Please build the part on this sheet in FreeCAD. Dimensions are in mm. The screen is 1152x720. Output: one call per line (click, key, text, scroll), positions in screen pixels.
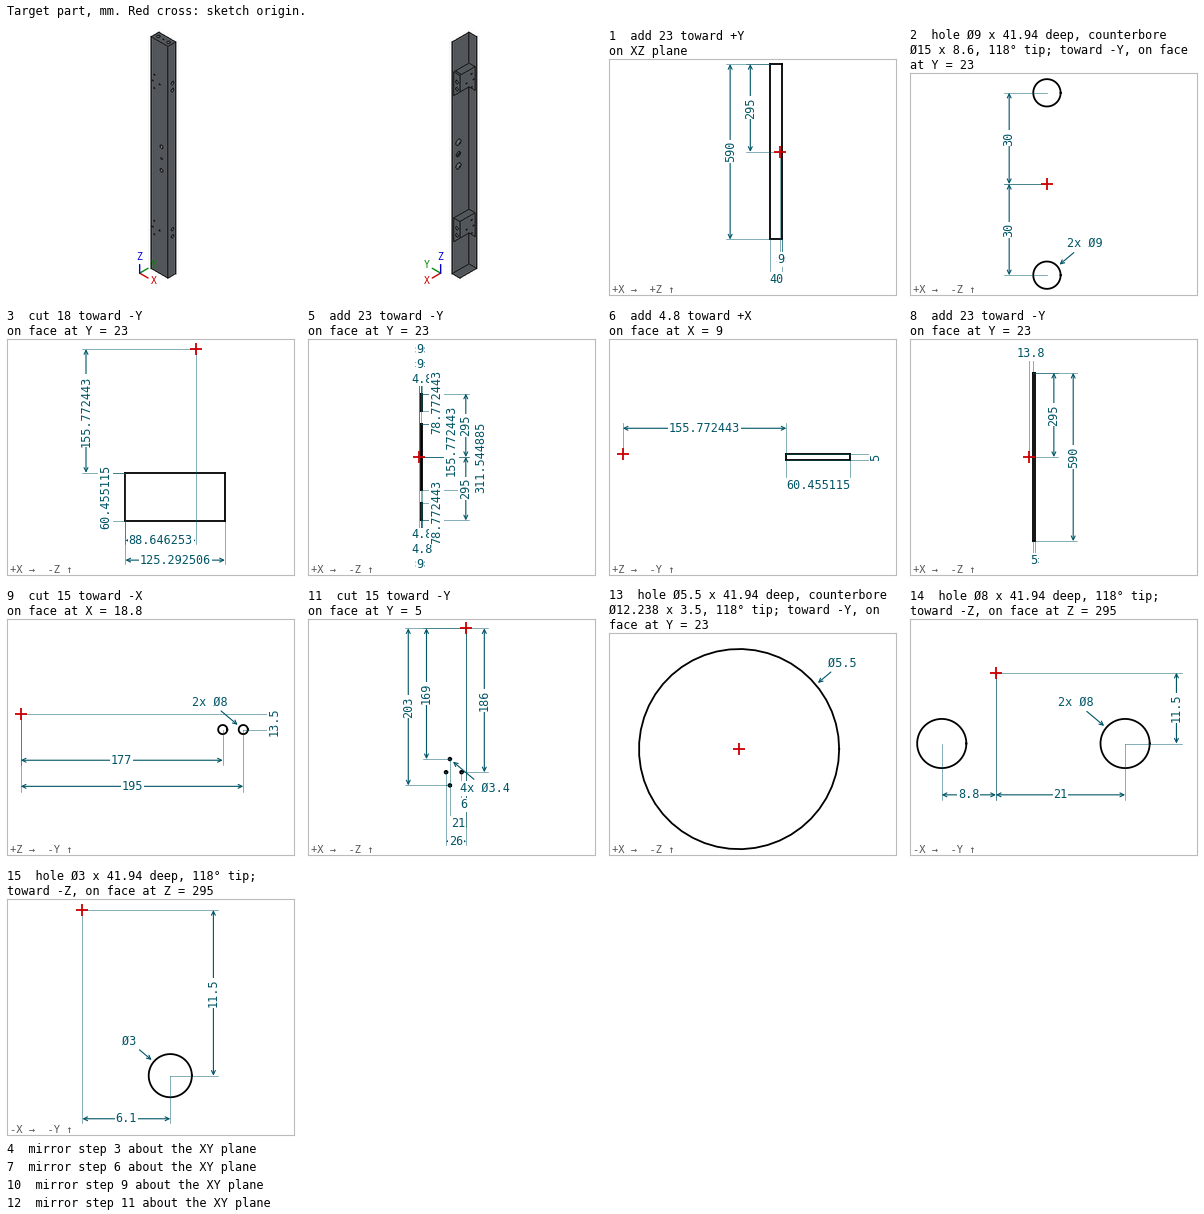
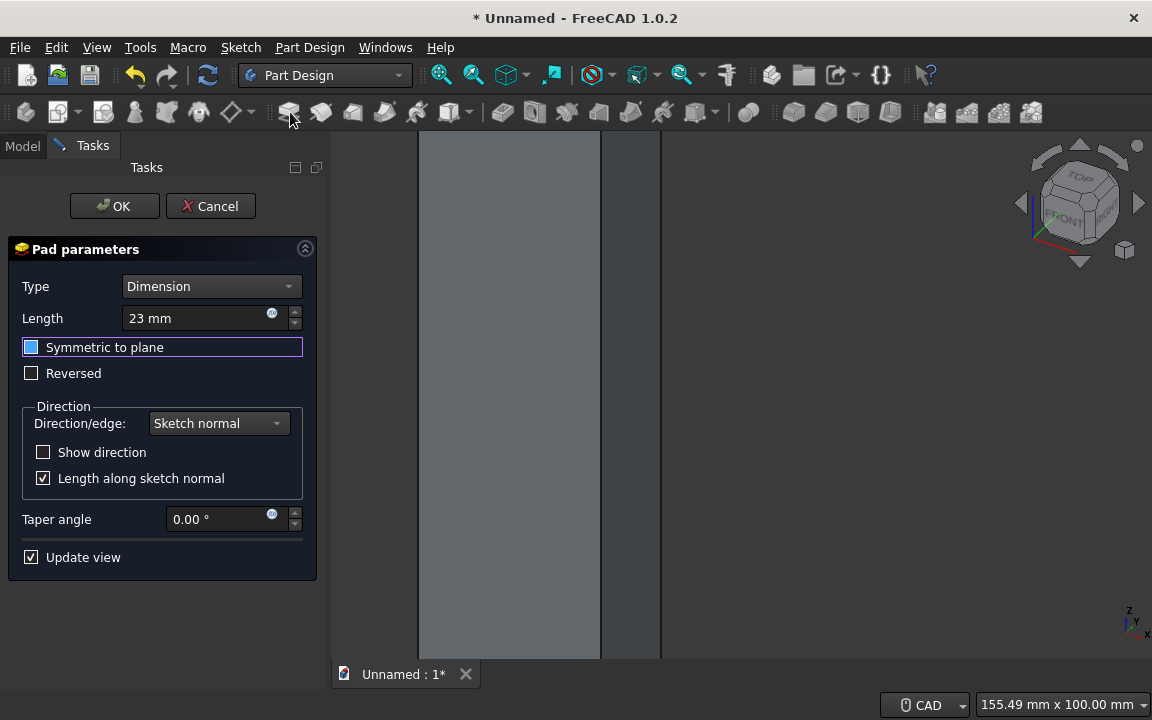
click(30, 373)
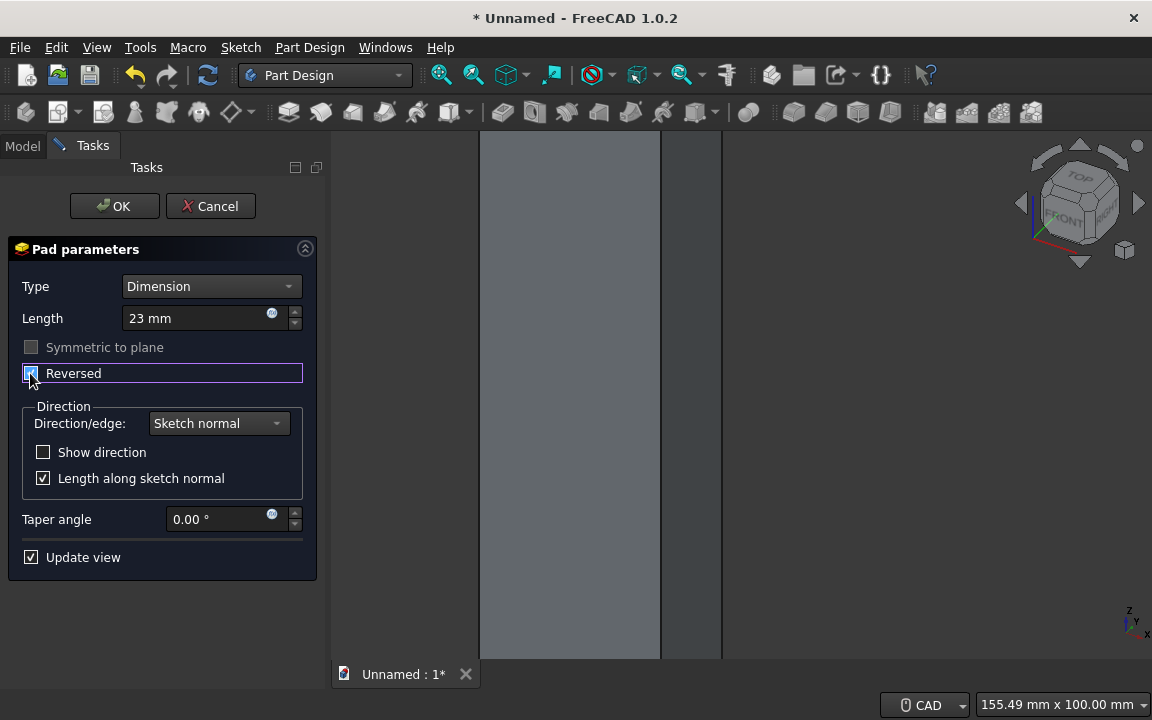
click(115, 206)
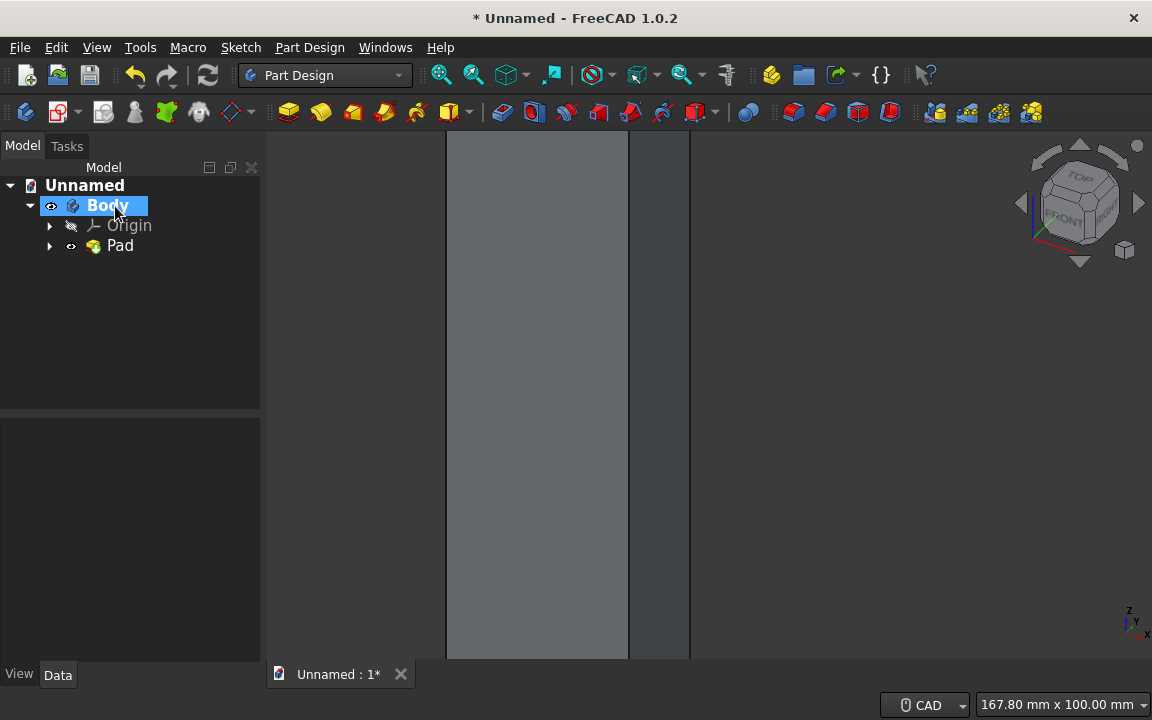
click(442, 76)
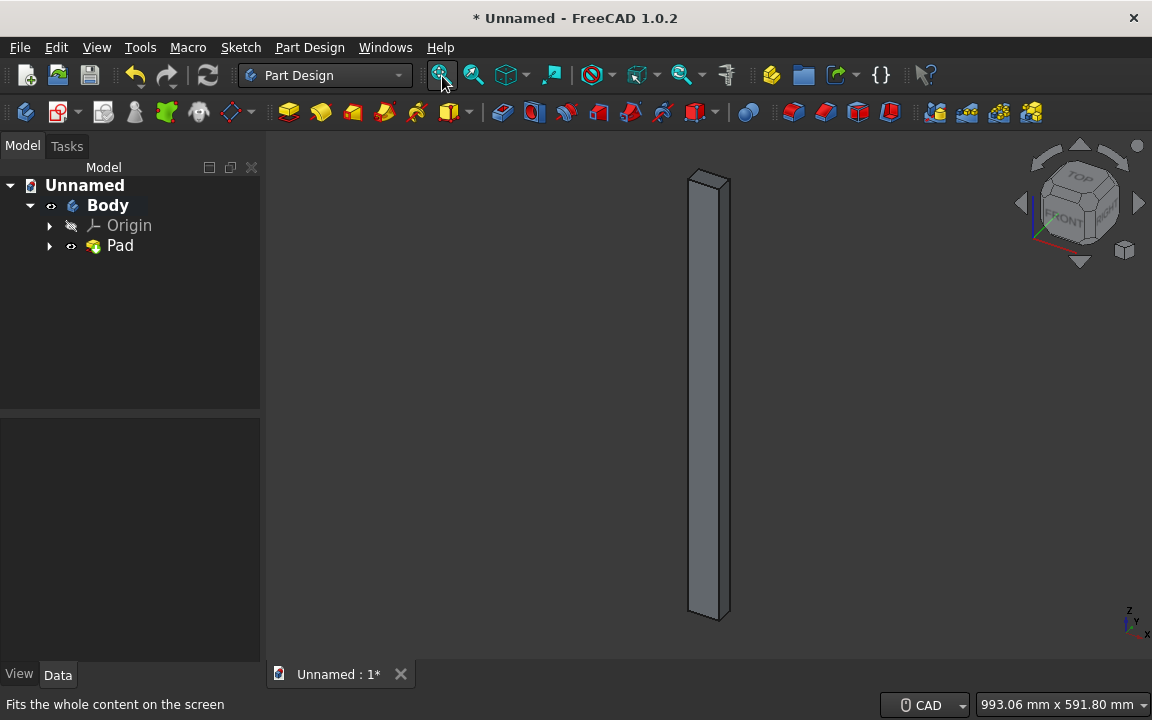
key(4)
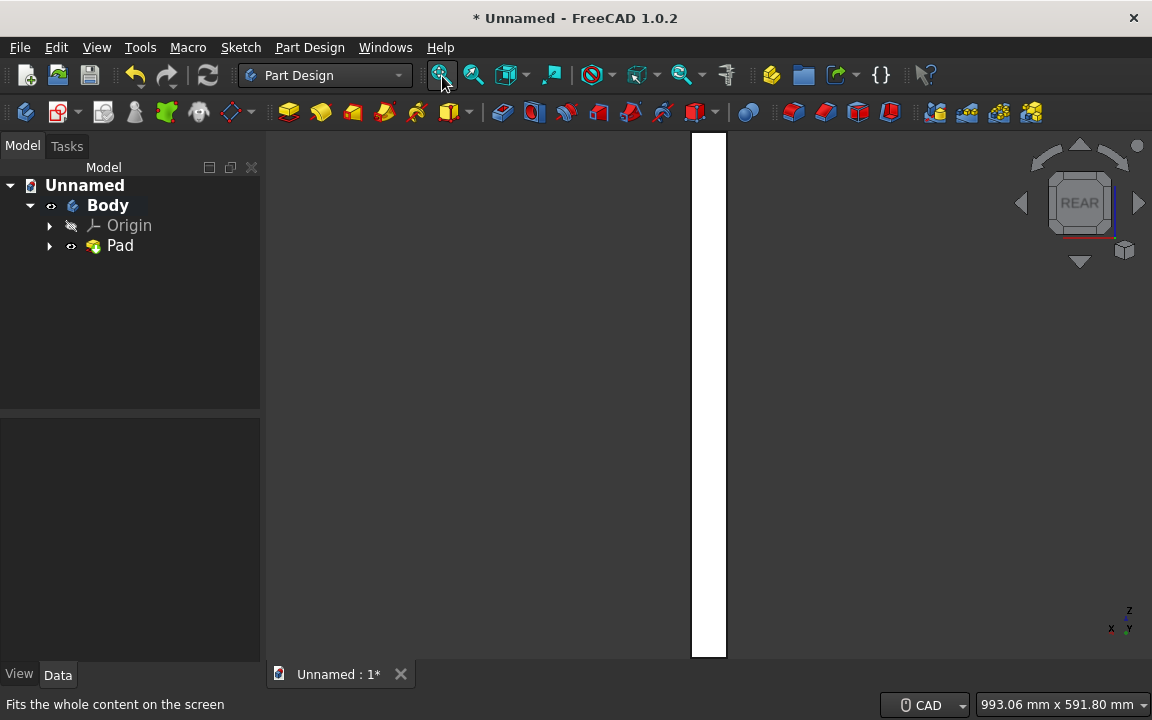
click(709, 168)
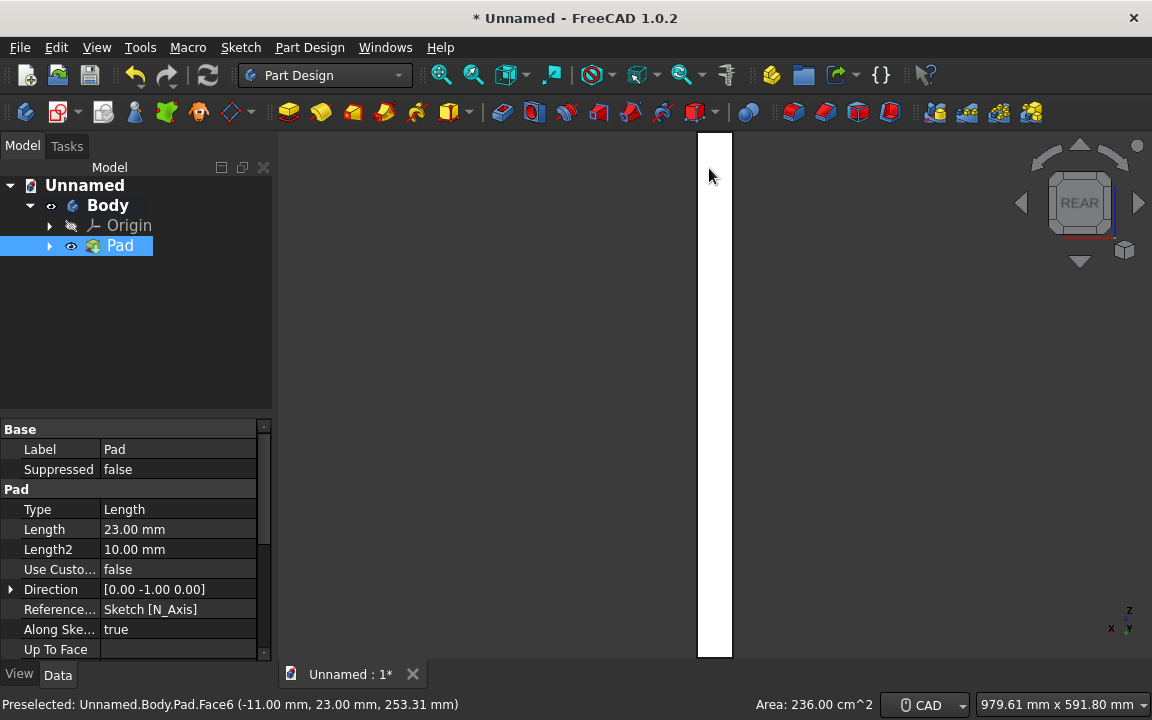
click(58, 112)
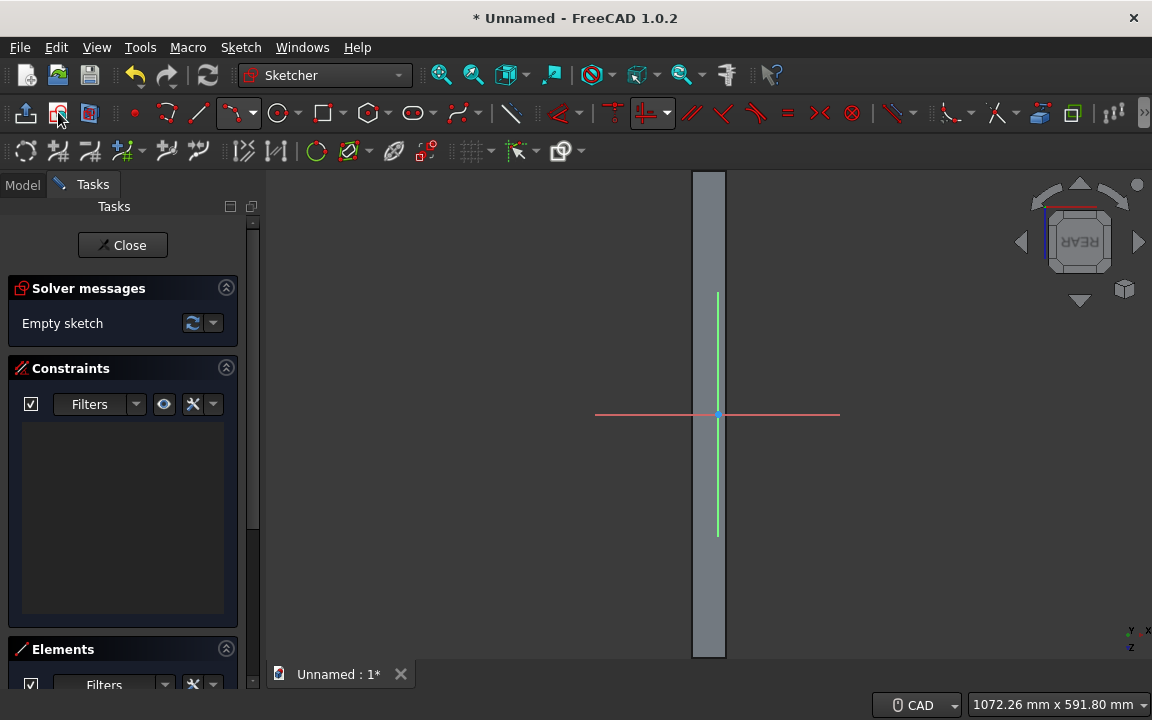
scroll(738, 415, up, 8)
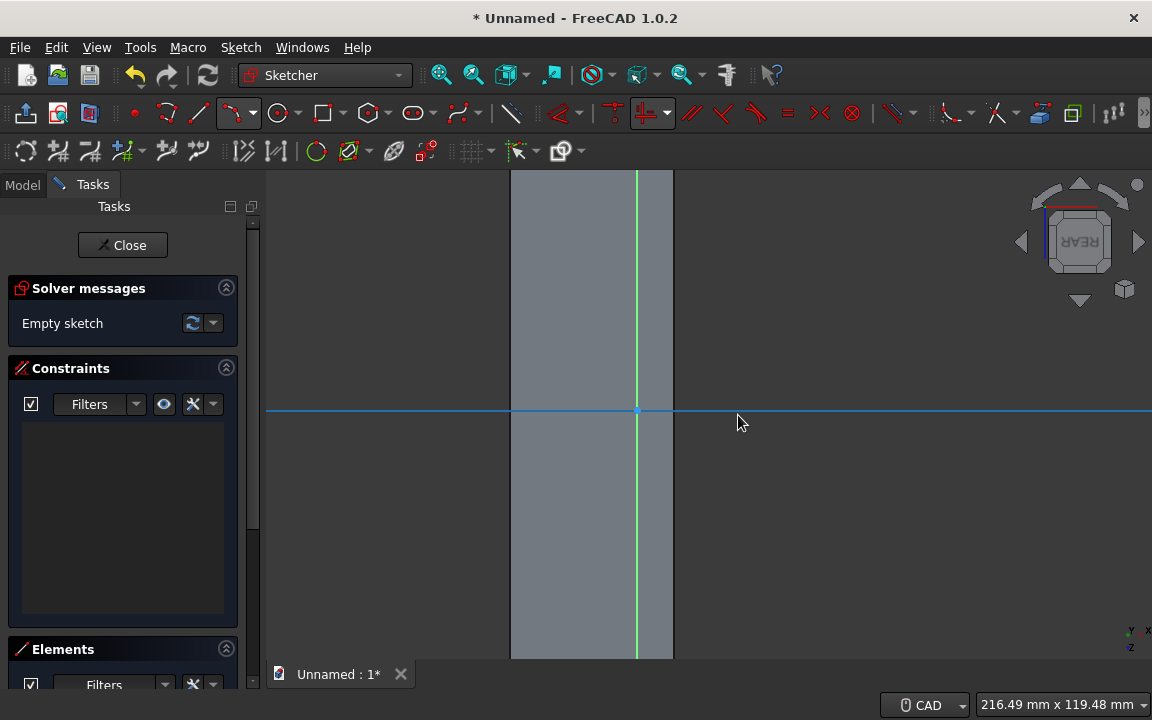
click(278, 114)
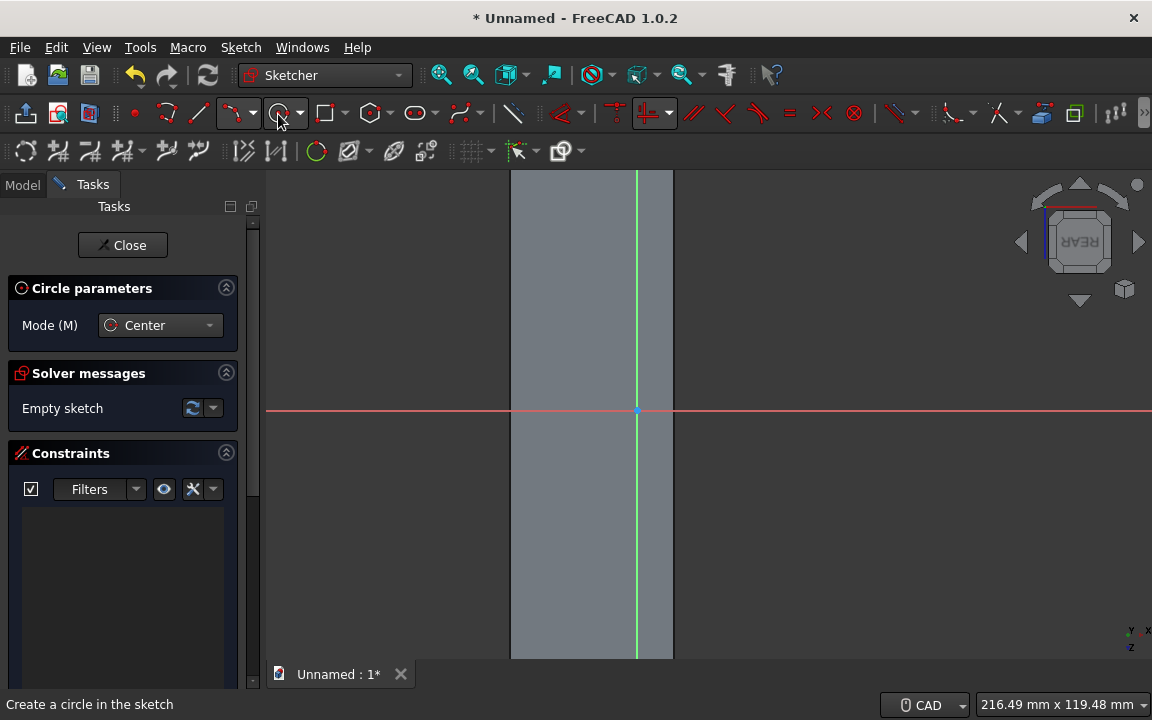
scroll(637, 533, up, 2)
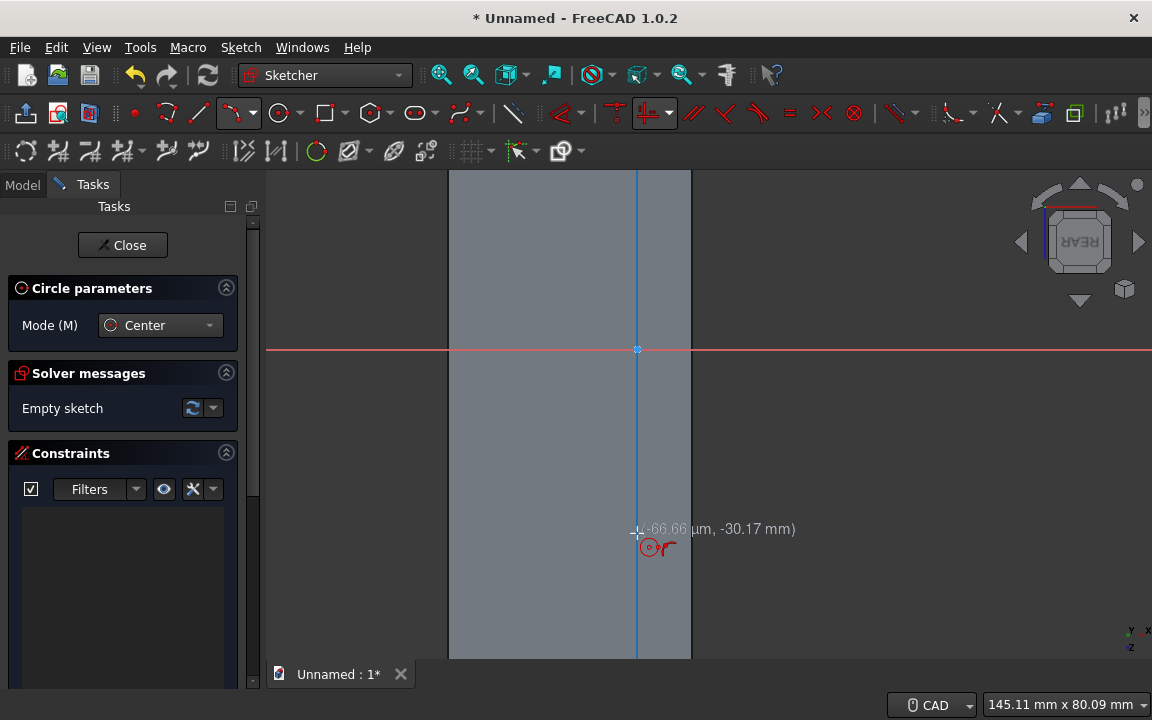
click(637, 533)
click(657, 514)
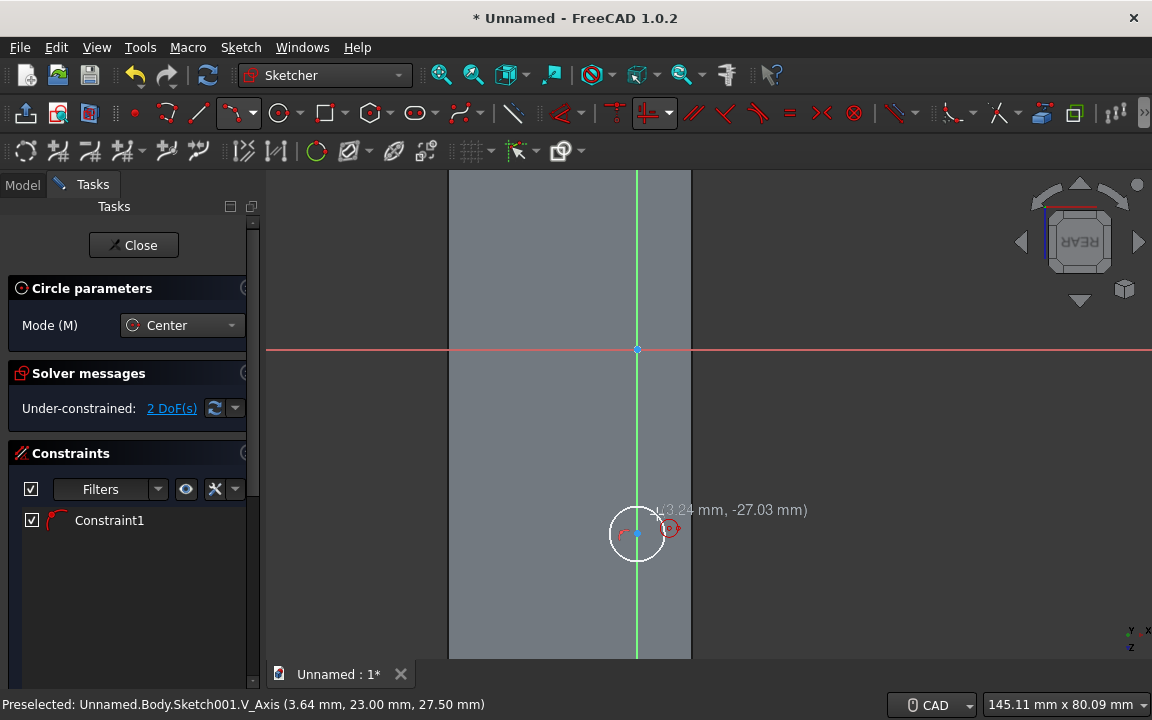
scroll(647, 546, down, 2)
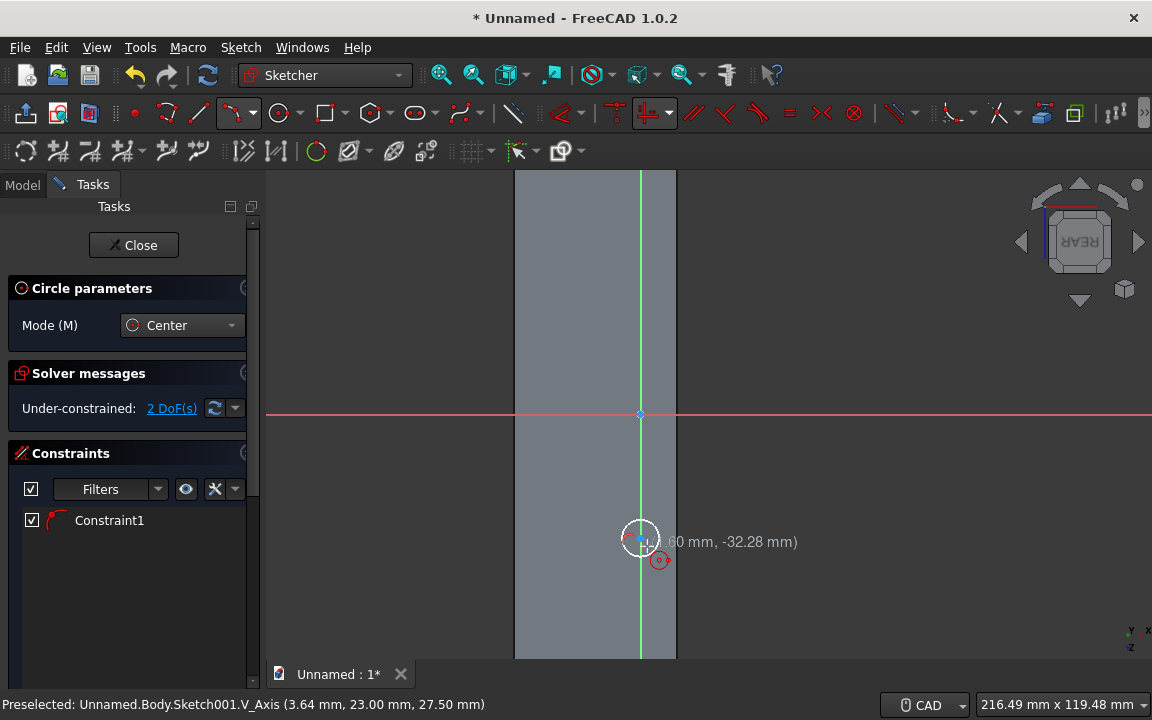
scroll(641, 292, up, 2)